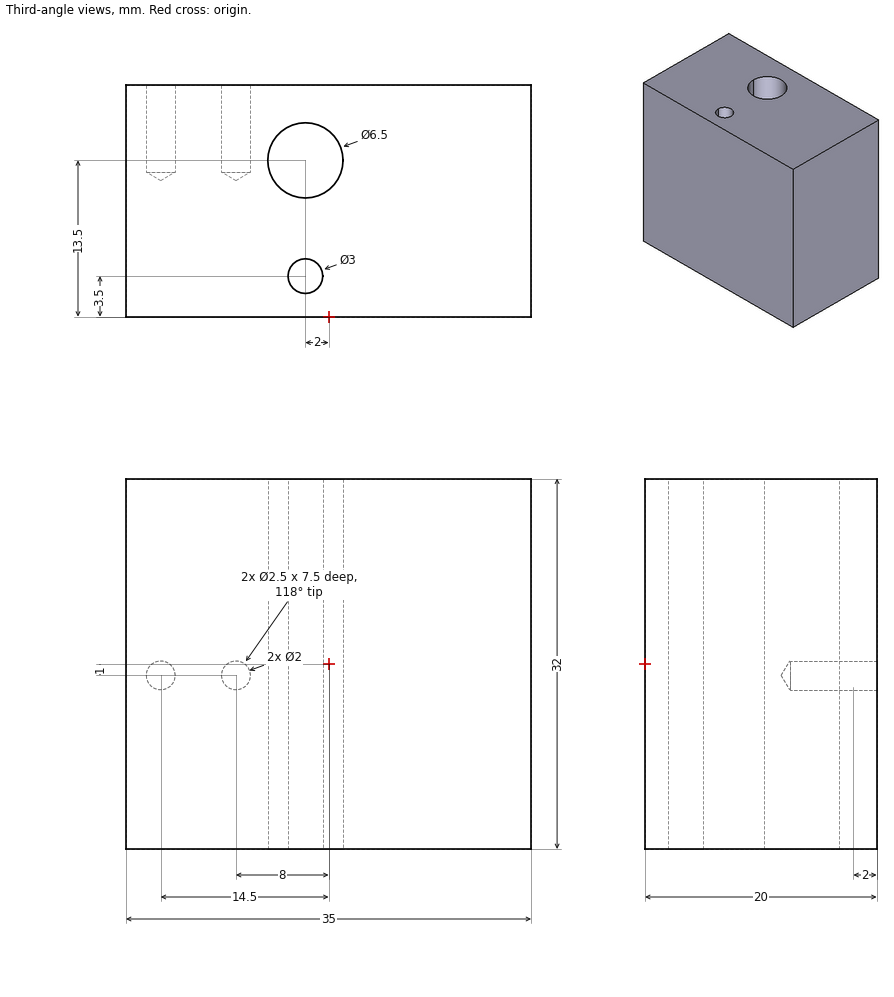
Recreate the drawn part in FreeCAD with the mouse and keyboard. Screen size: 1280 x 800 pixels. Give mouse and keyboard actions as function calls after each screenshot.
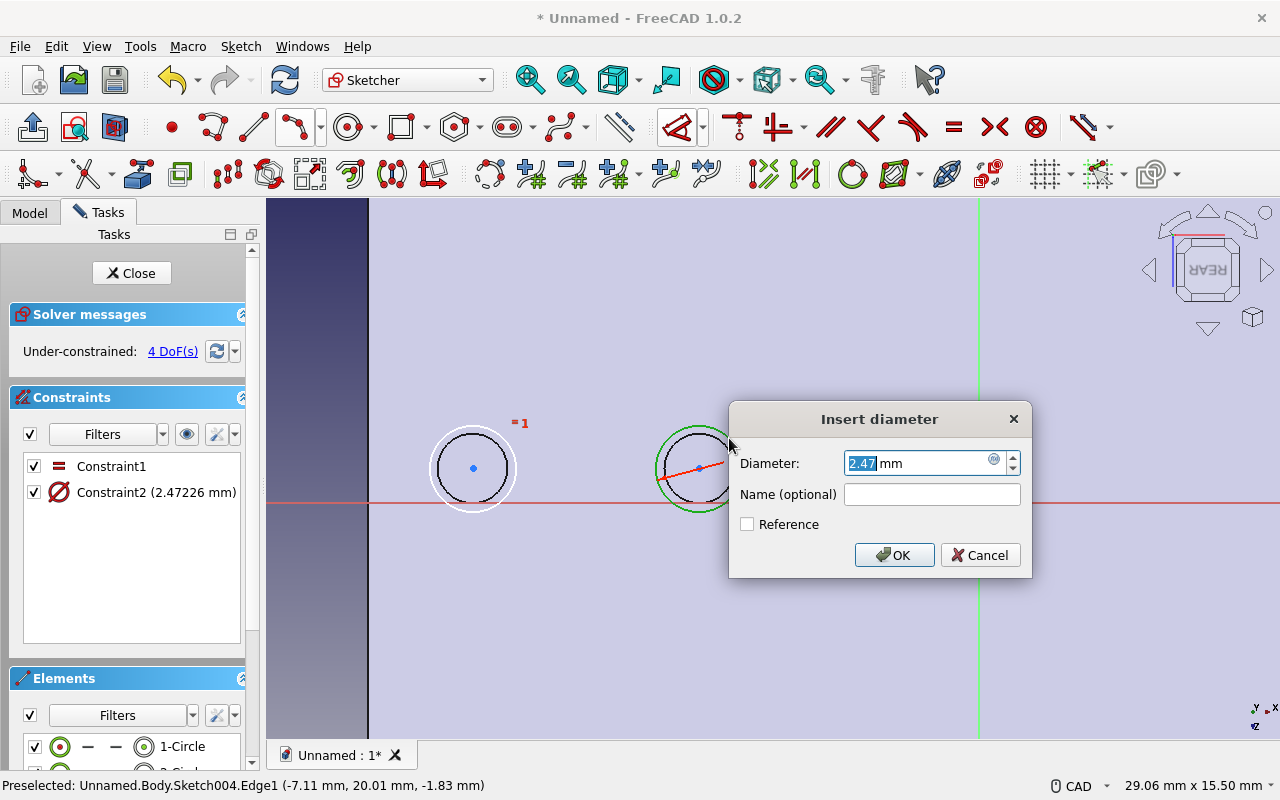
text(2.5)
key(Return)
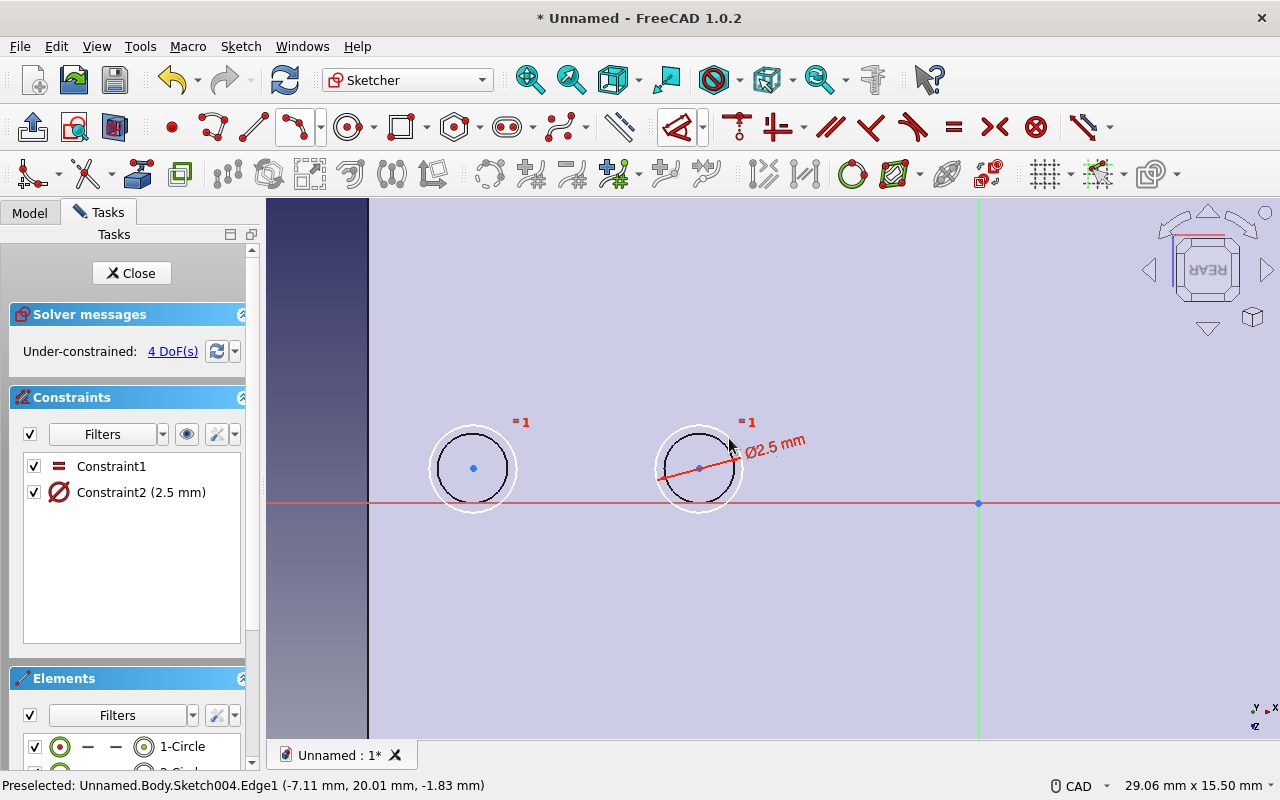
click(699, 469)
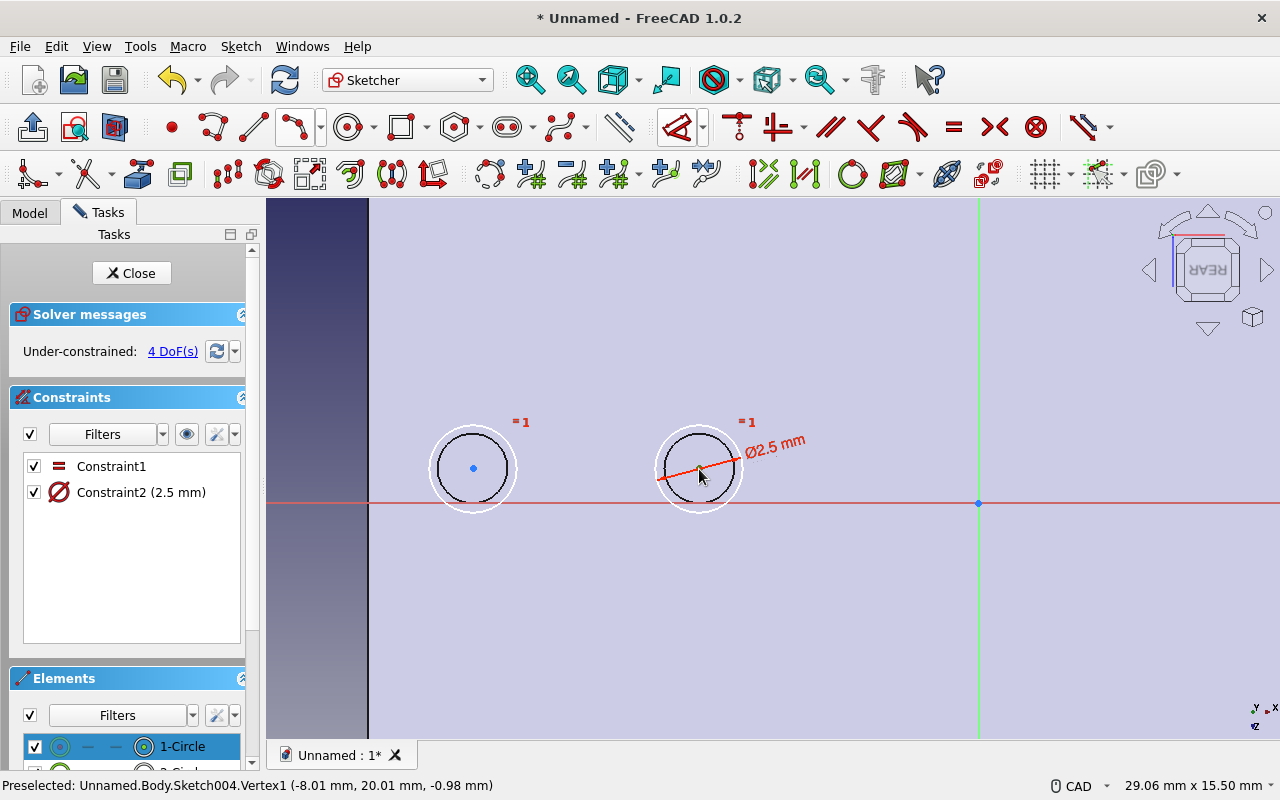
click(702, 128)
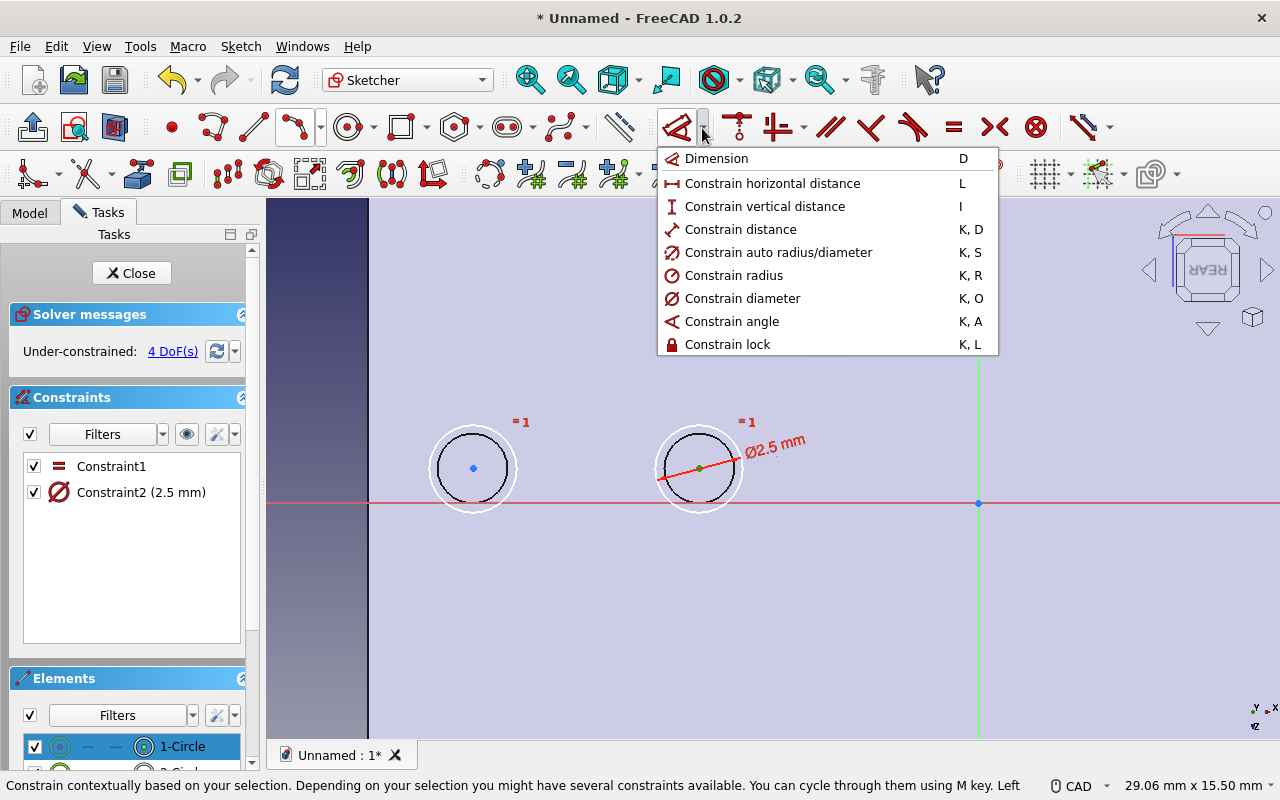
click(828, 184)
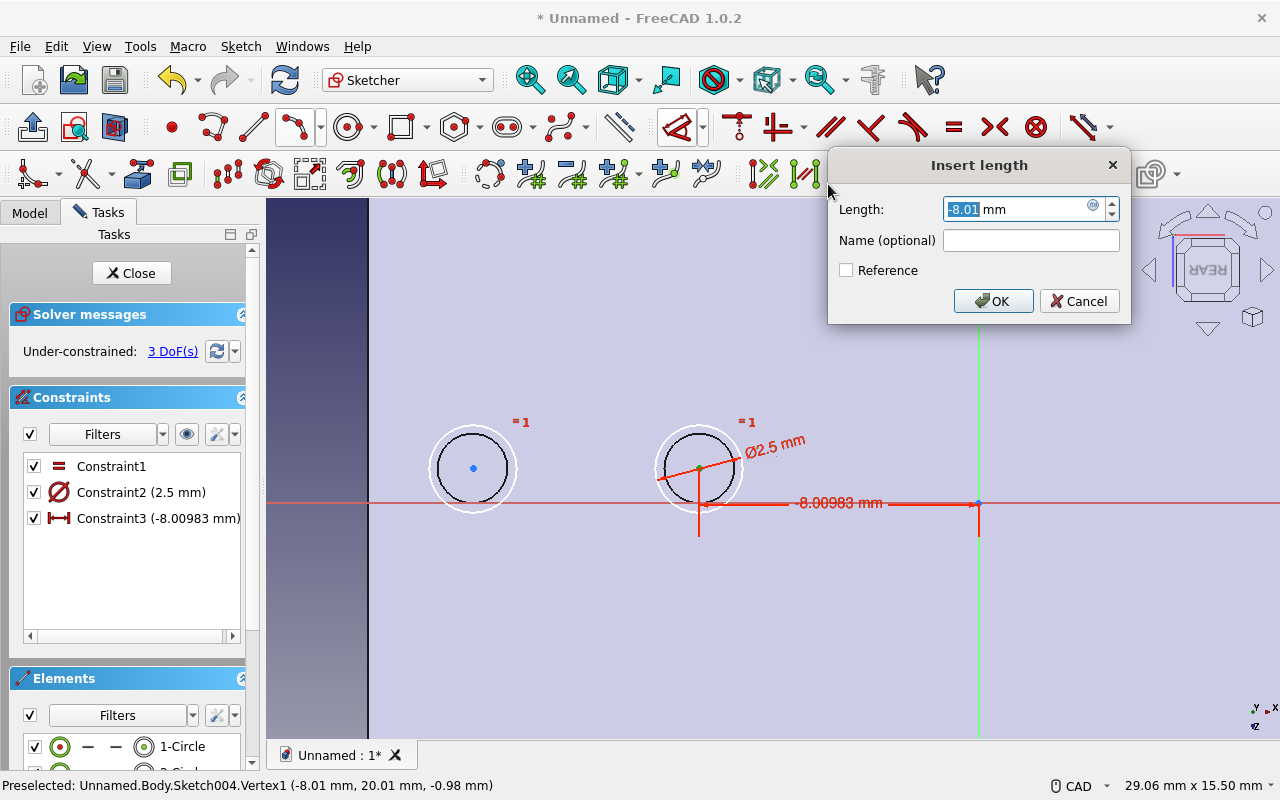
text(-8)
key(Return)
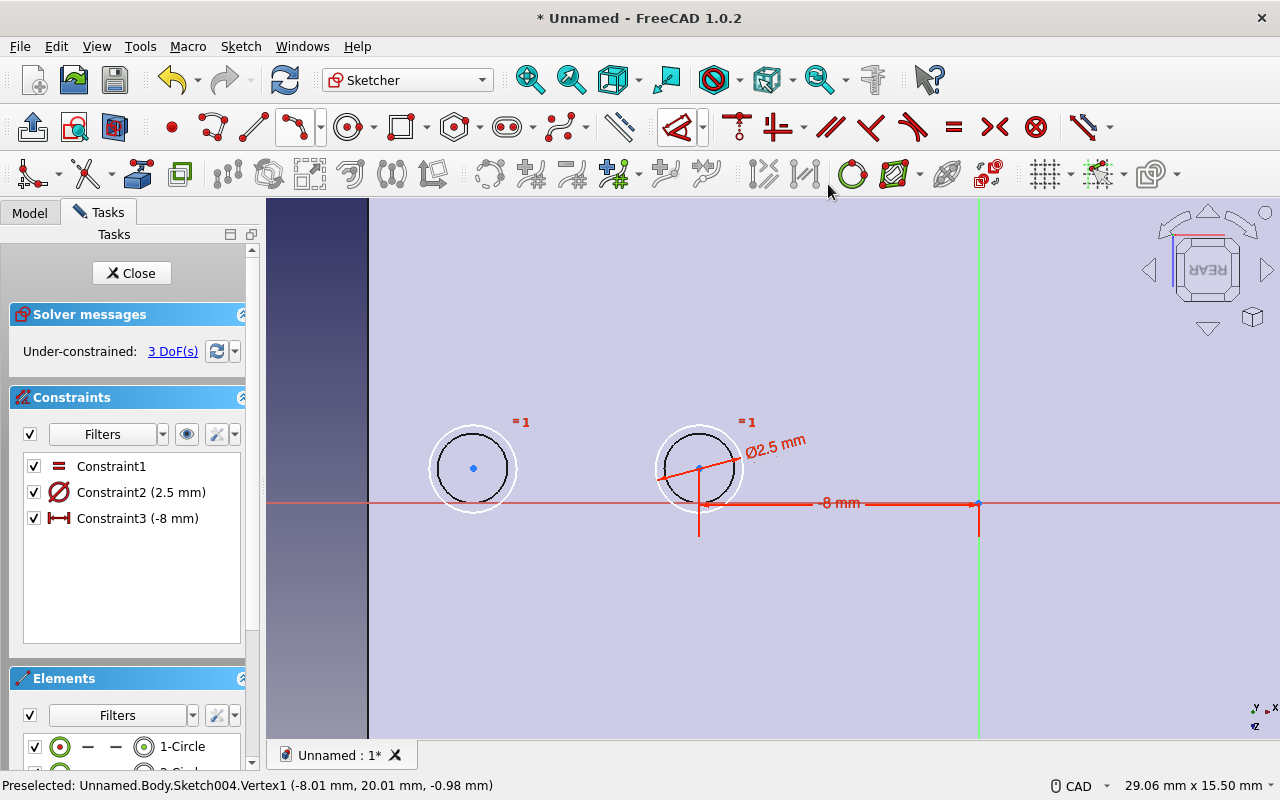
click(699, 469)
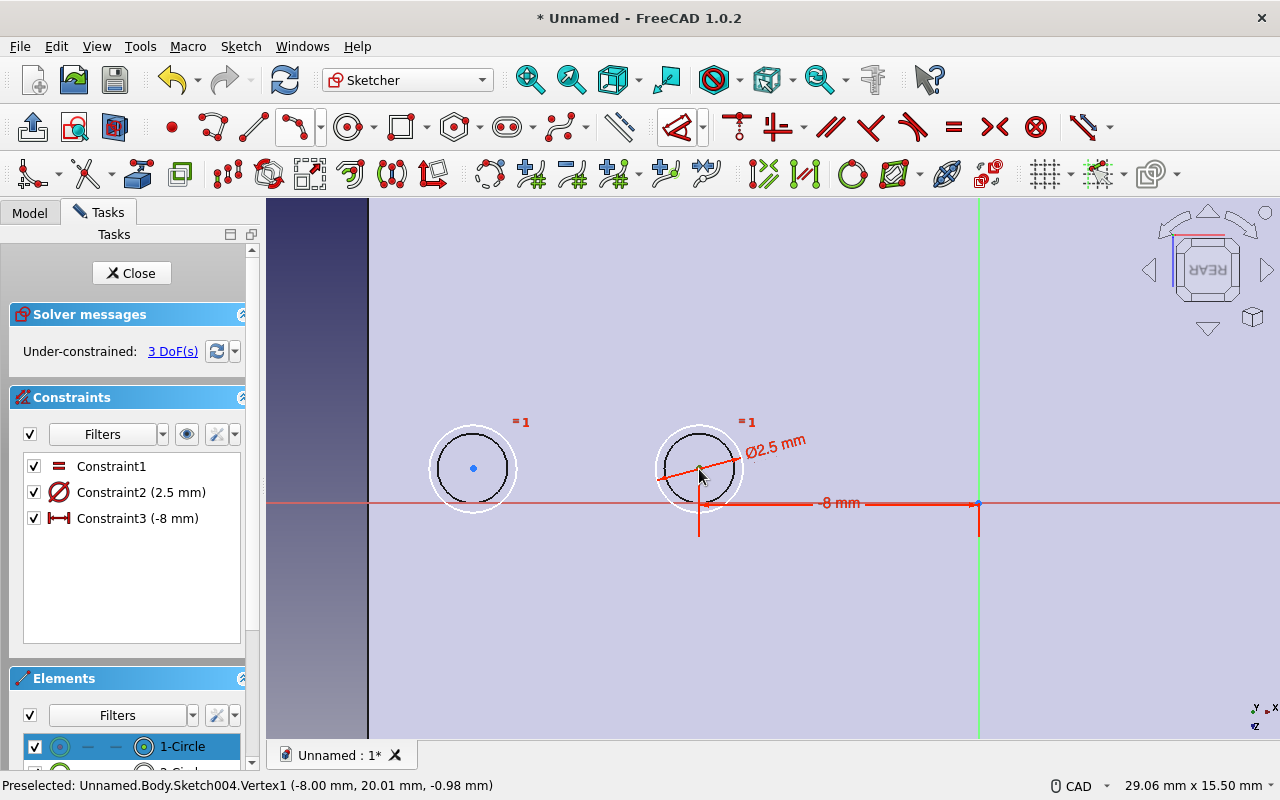
key(i)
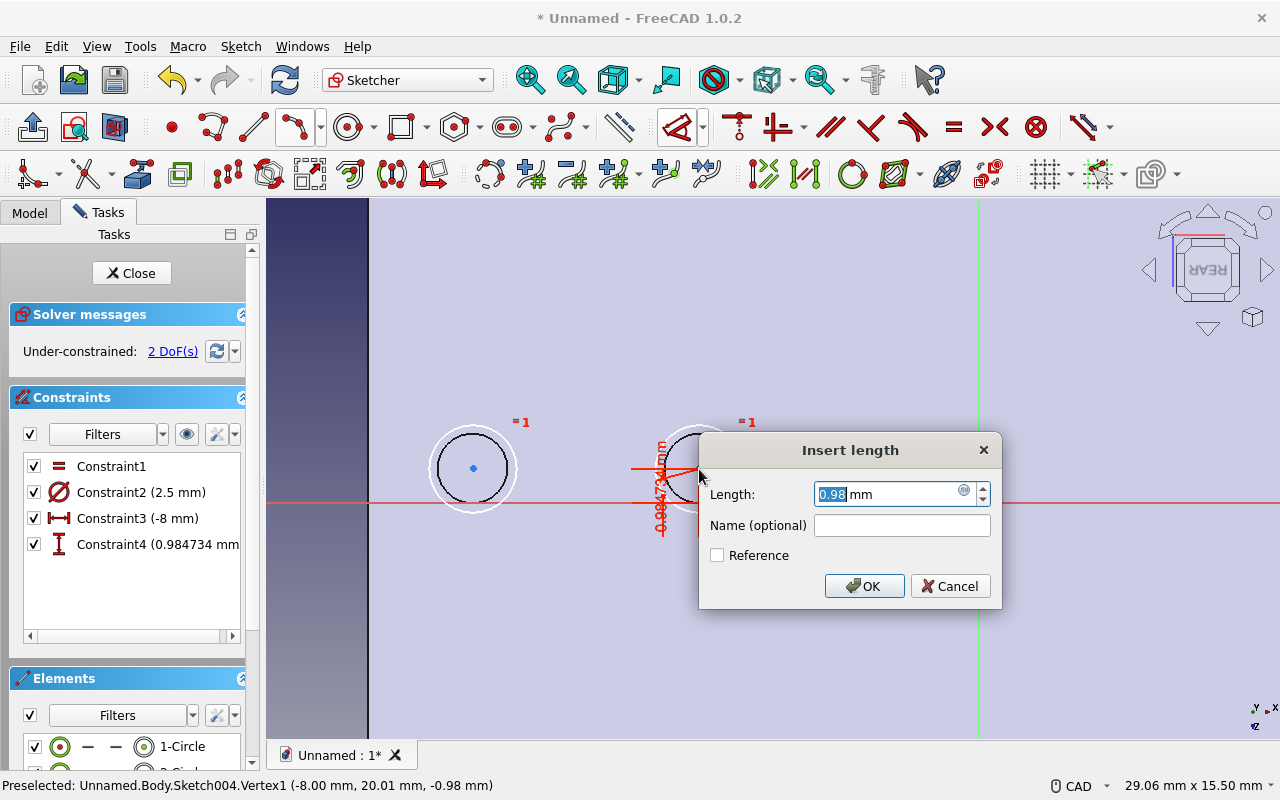
text(1)
key(Return)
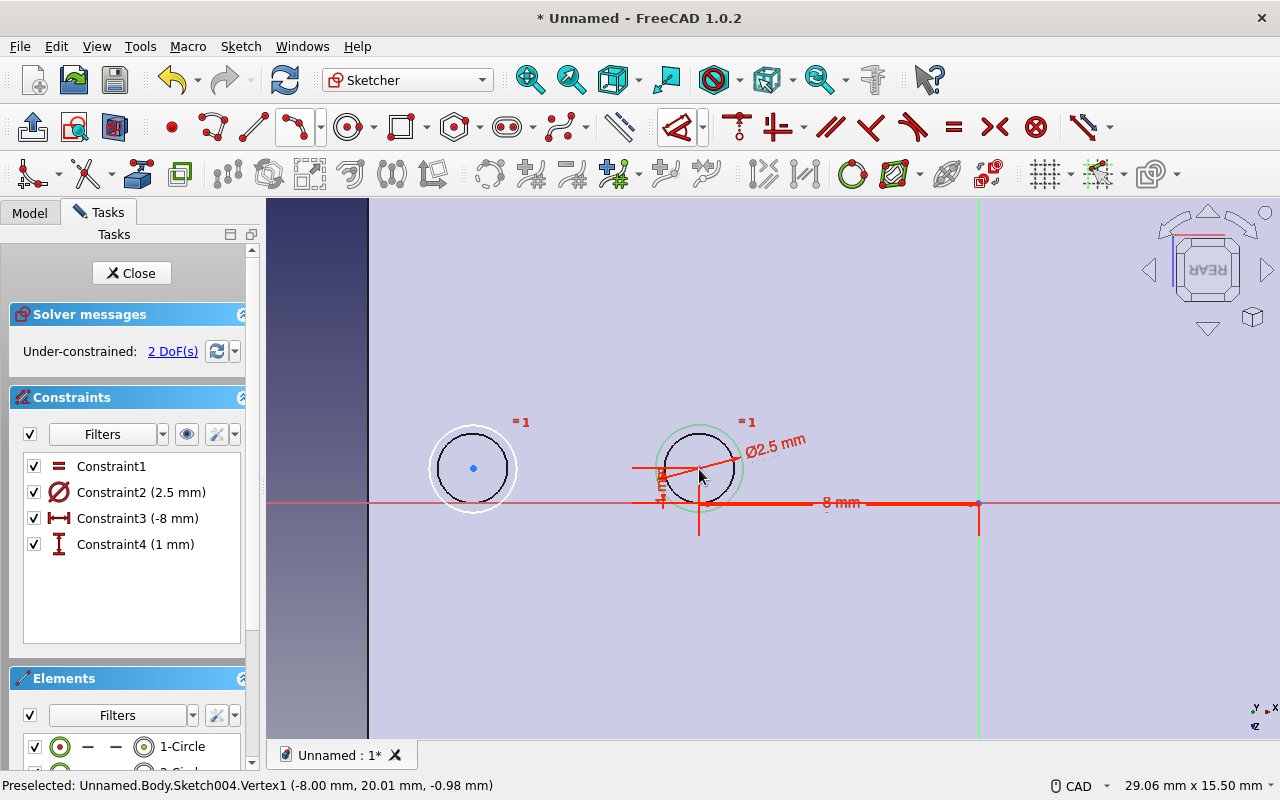
click(473, 469)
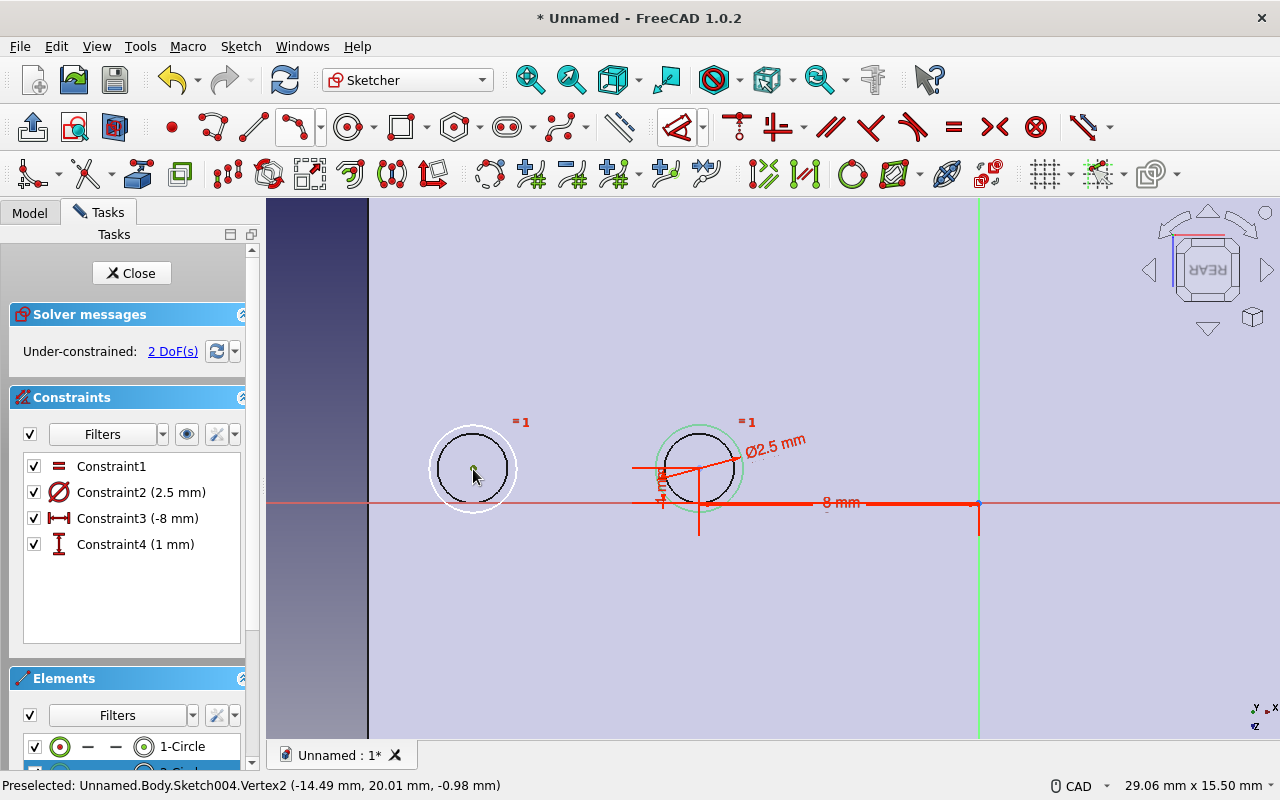
click(702, 128)